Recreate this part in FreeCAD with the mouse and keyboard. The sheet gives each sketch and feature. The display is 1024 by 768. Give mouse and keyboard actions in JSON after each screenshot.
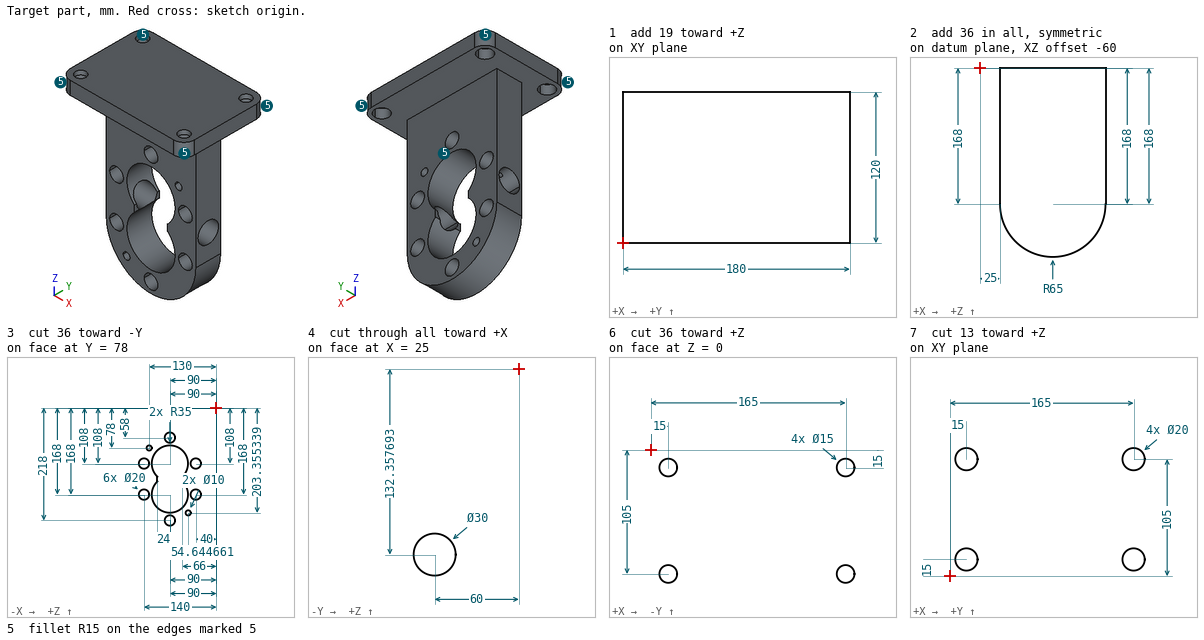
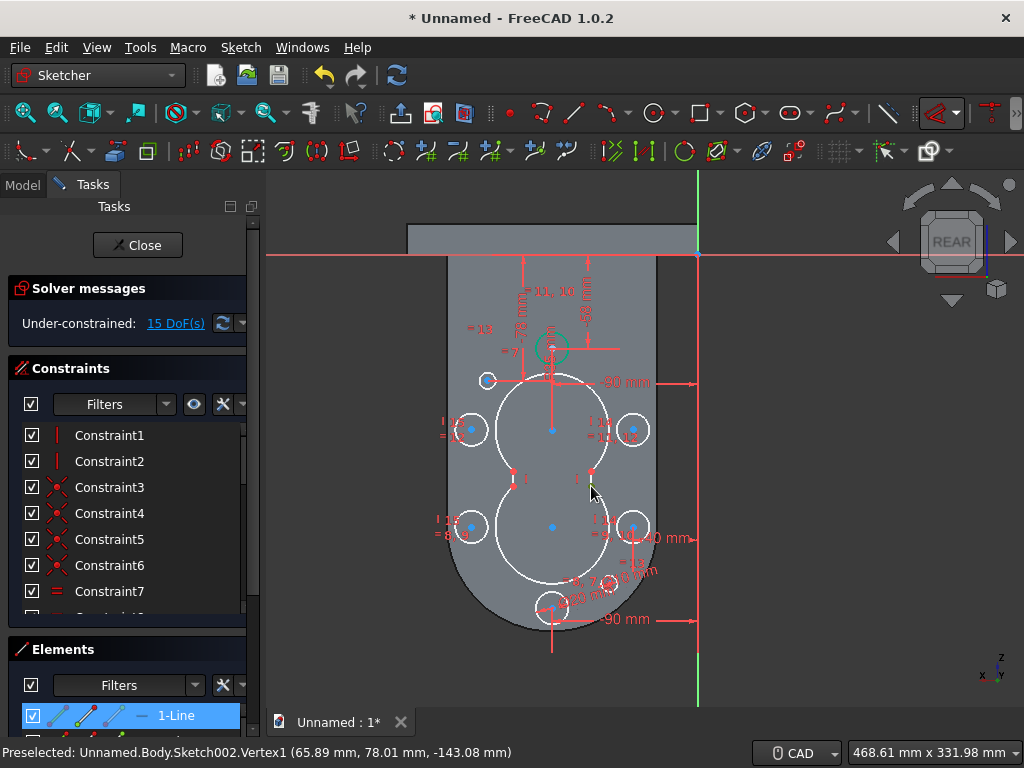
{"action": "left_click", "coordinate": [958, 114]}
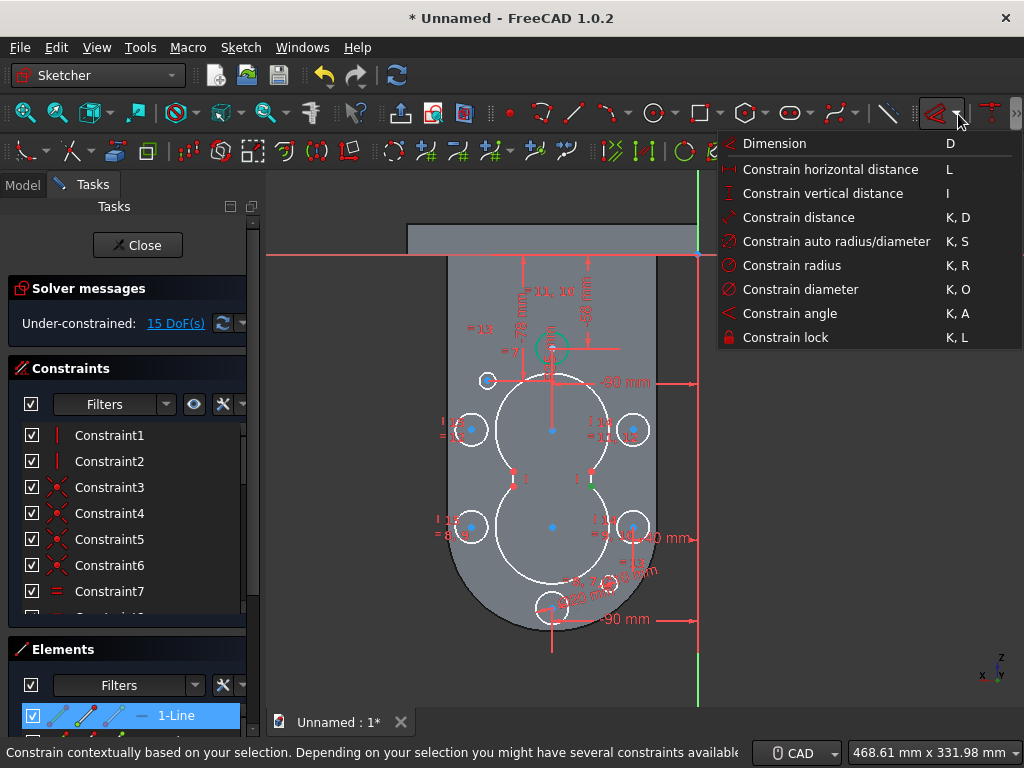
{"action": "left_click", "coordinate": [870, 169]}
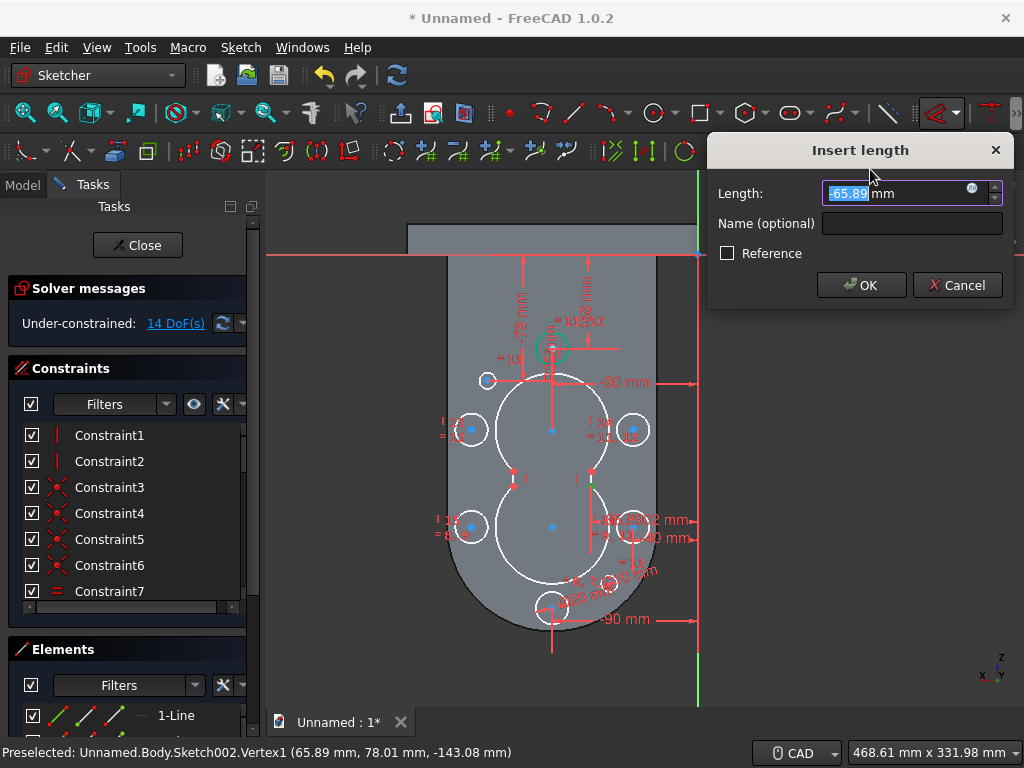
{"action": "type", "text": "-66"}
{"action": "key", "text": "Return"}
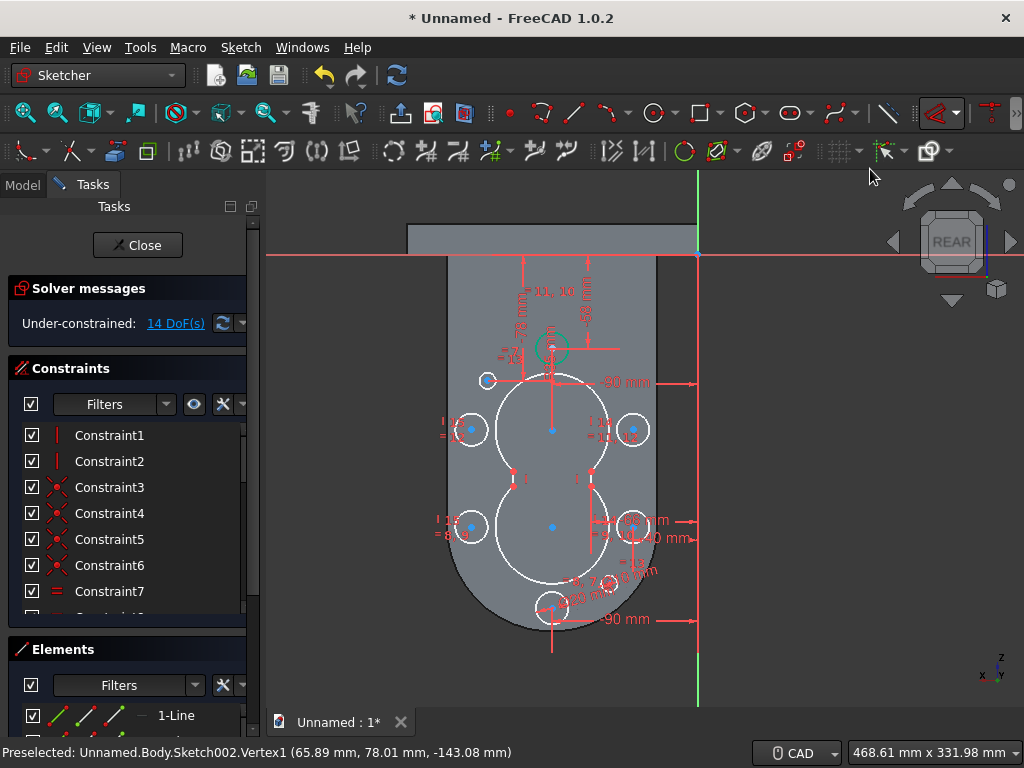
{"action": "left_click", "coordinate": [552, 430]}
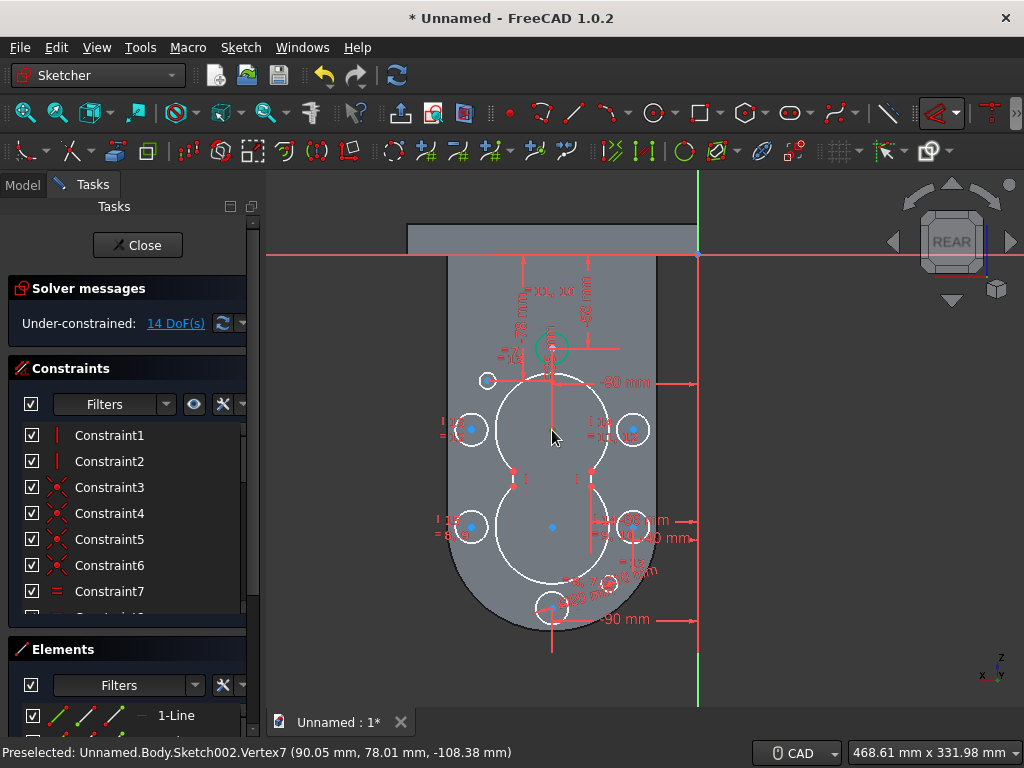
{"action": "left_click", "coordinate": [958, 114]}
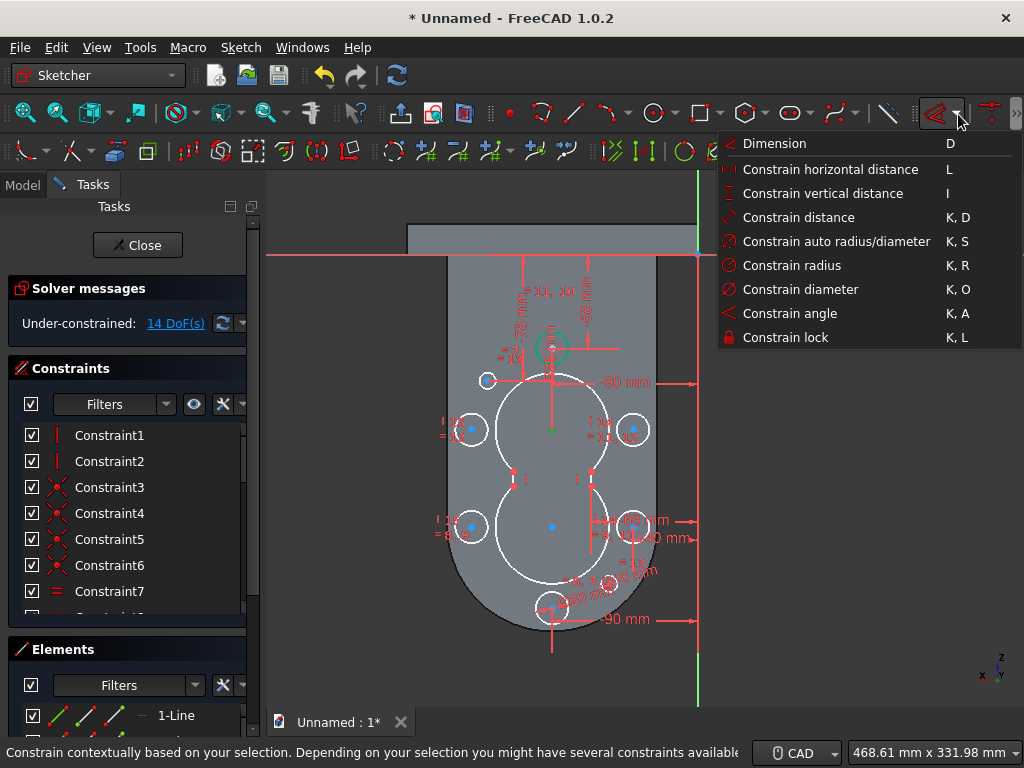
{"action": "left_click", "coordinate": [870, 169]}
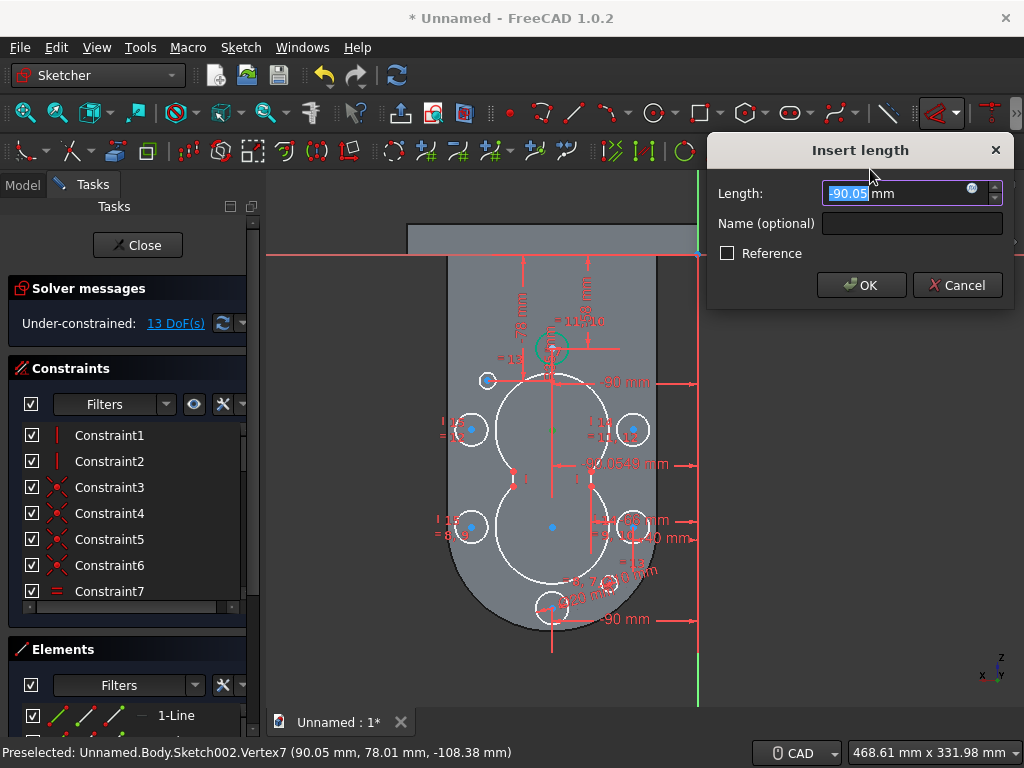
{"action": "type", "text": "-90"}
{"action": "key", "text": "Return"}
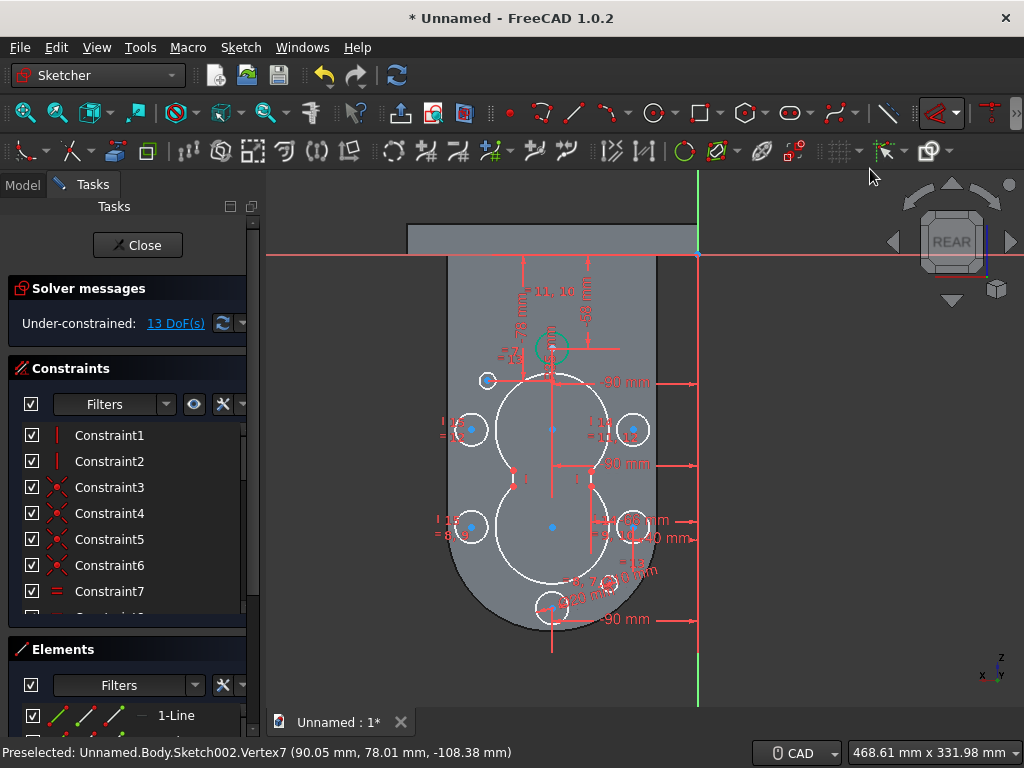
{"action": "left_click", "coordinate": [552, 527]}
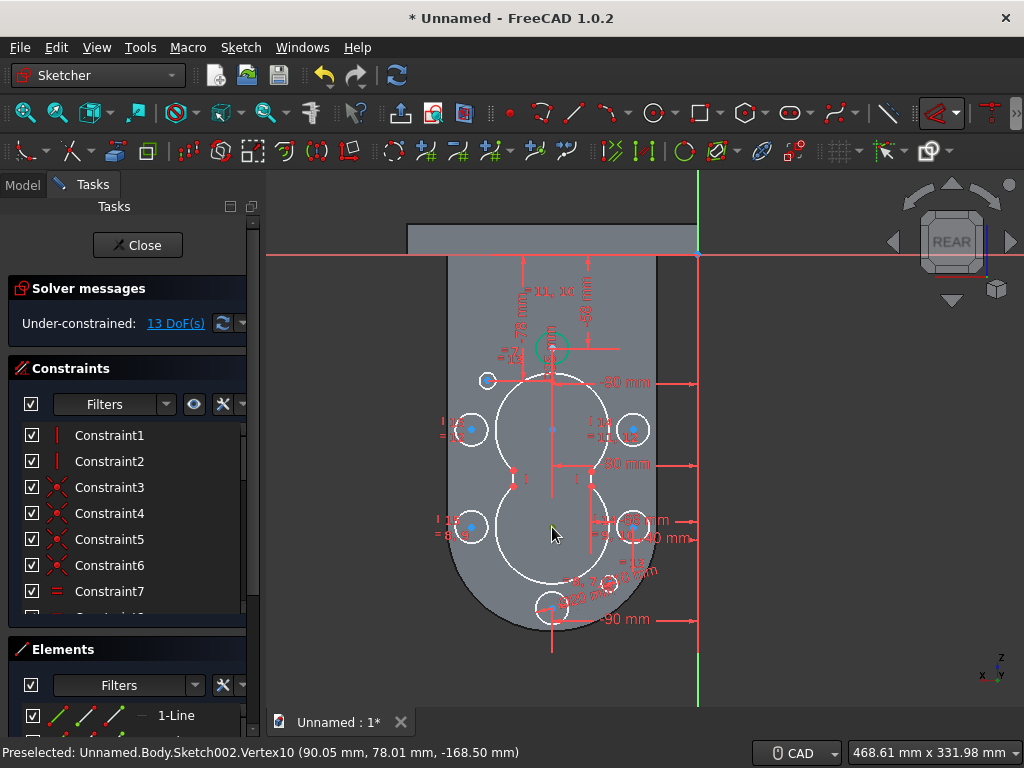
{"action": "key", "text": "l"}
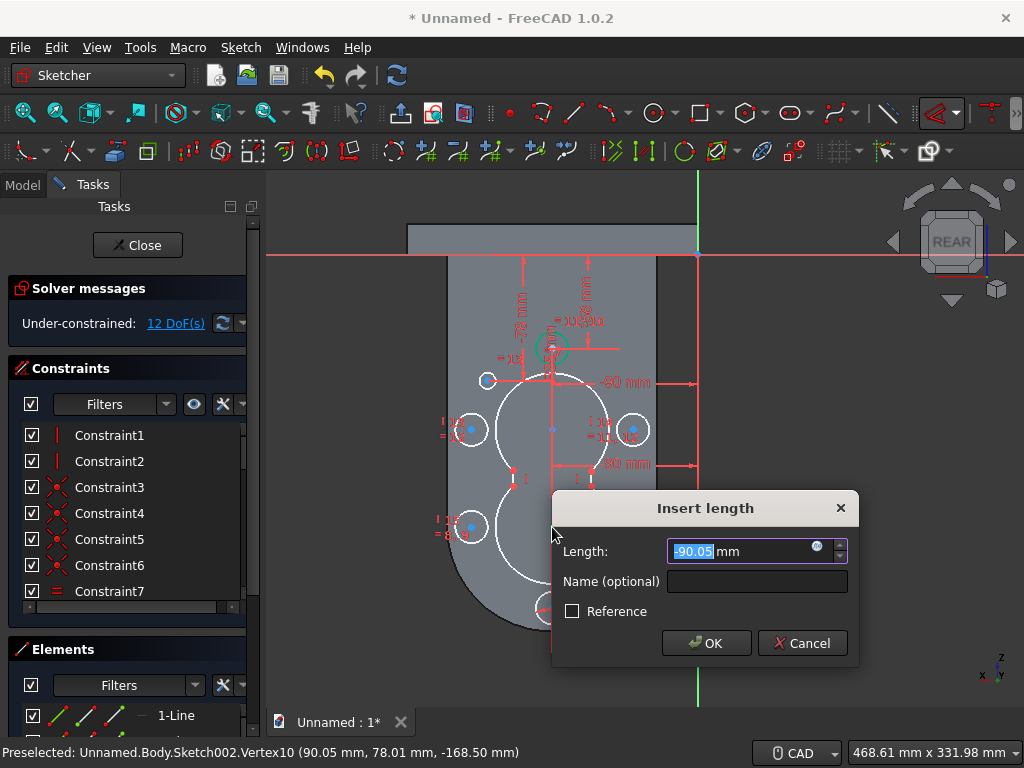
{"action": "type", "text": "-90"}
{"action": "key", "text": "Return"}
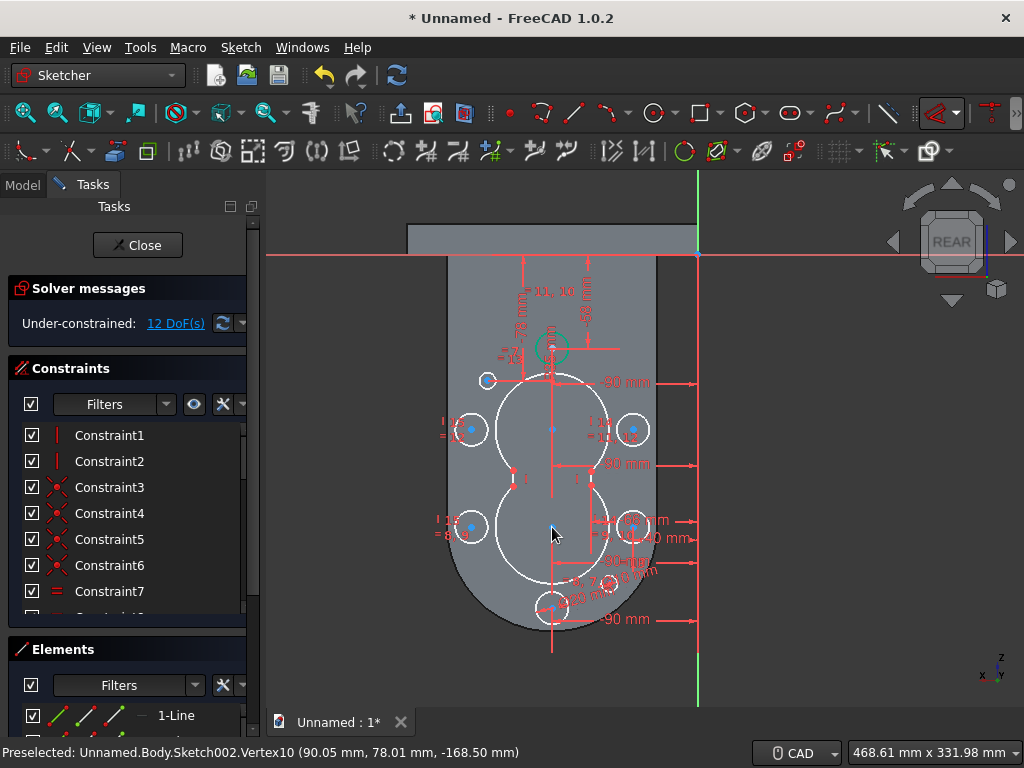
{"action": "left_click", "coordinate": [552, 608]}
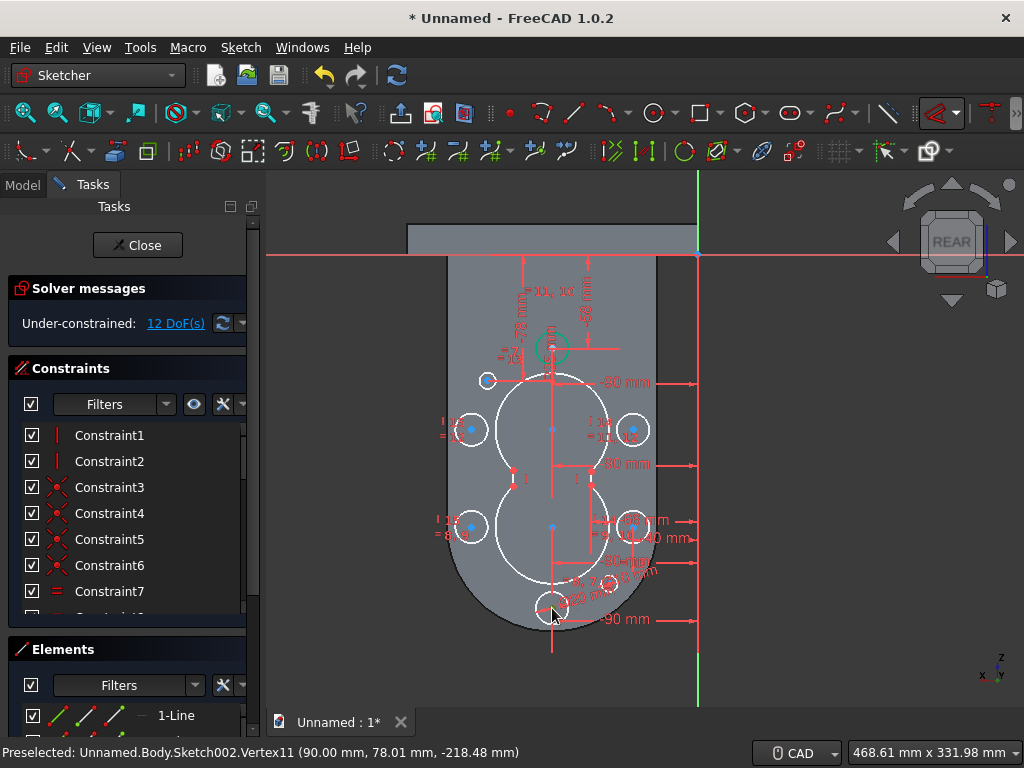
{"action": "left_click", "coordinate": [958, 114]}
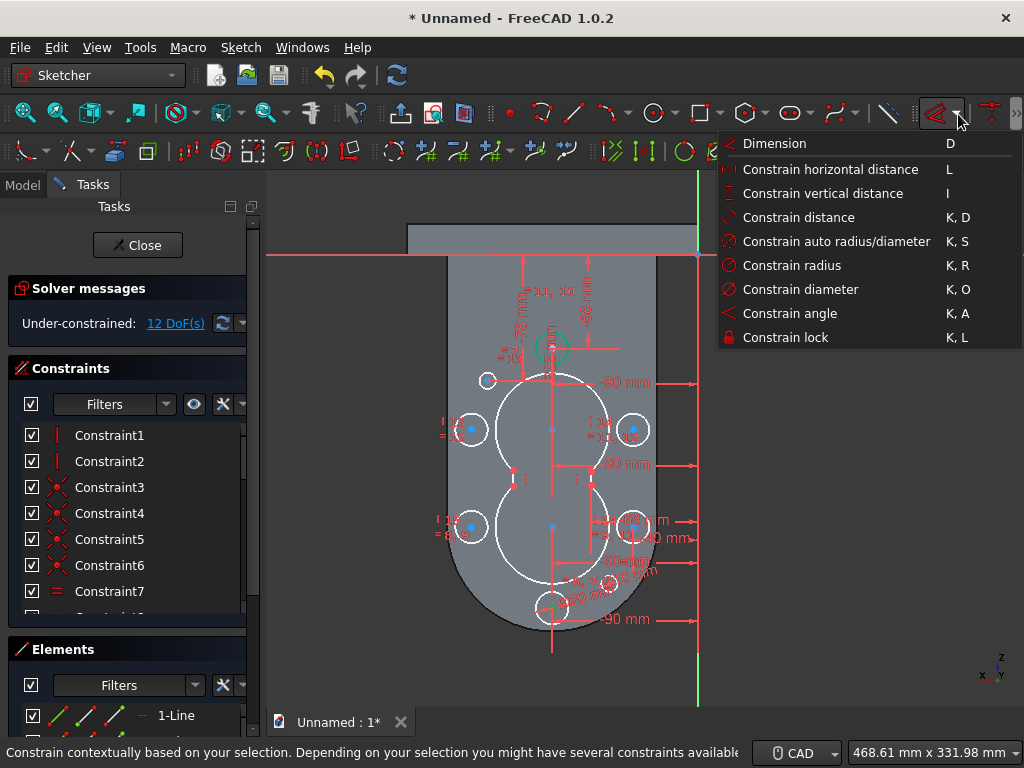
{"action": "left_click", "coordinate": [870, 193]}